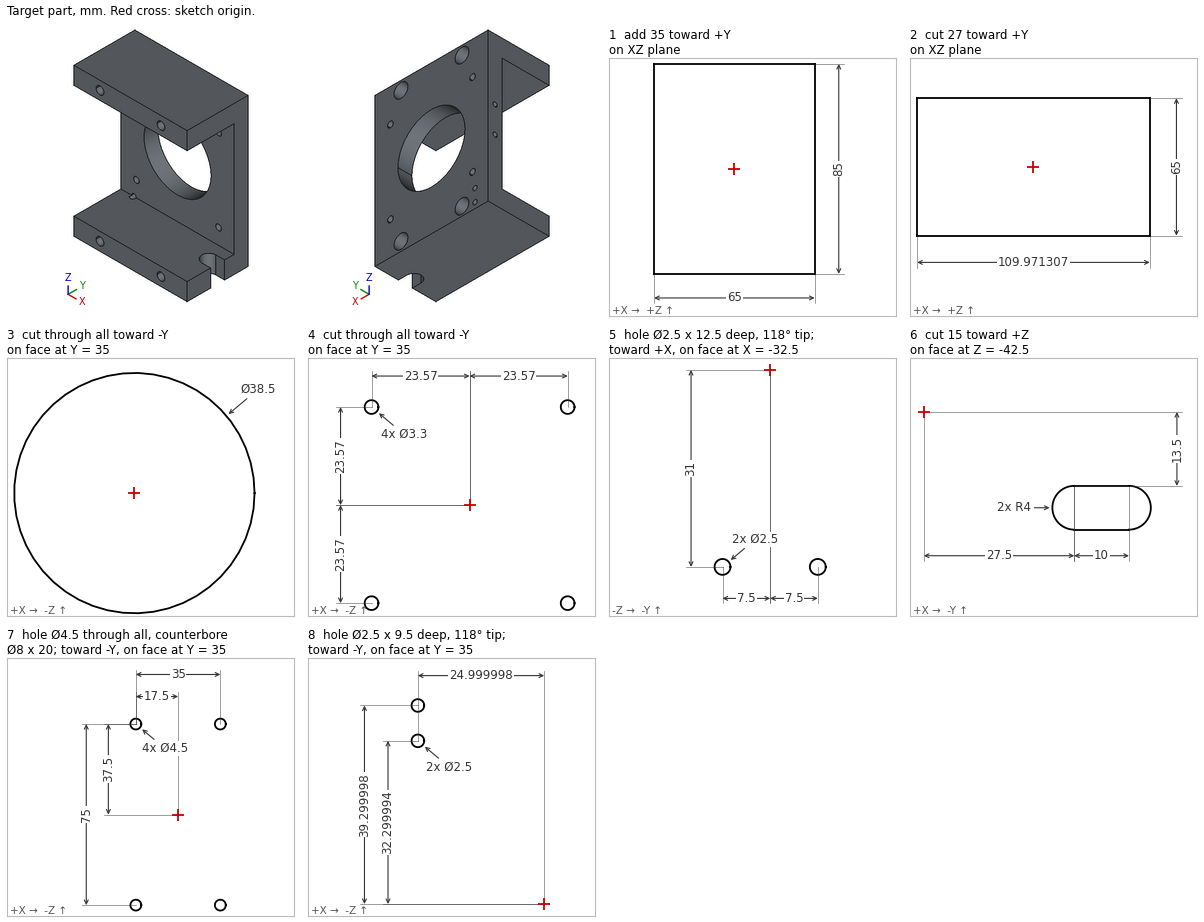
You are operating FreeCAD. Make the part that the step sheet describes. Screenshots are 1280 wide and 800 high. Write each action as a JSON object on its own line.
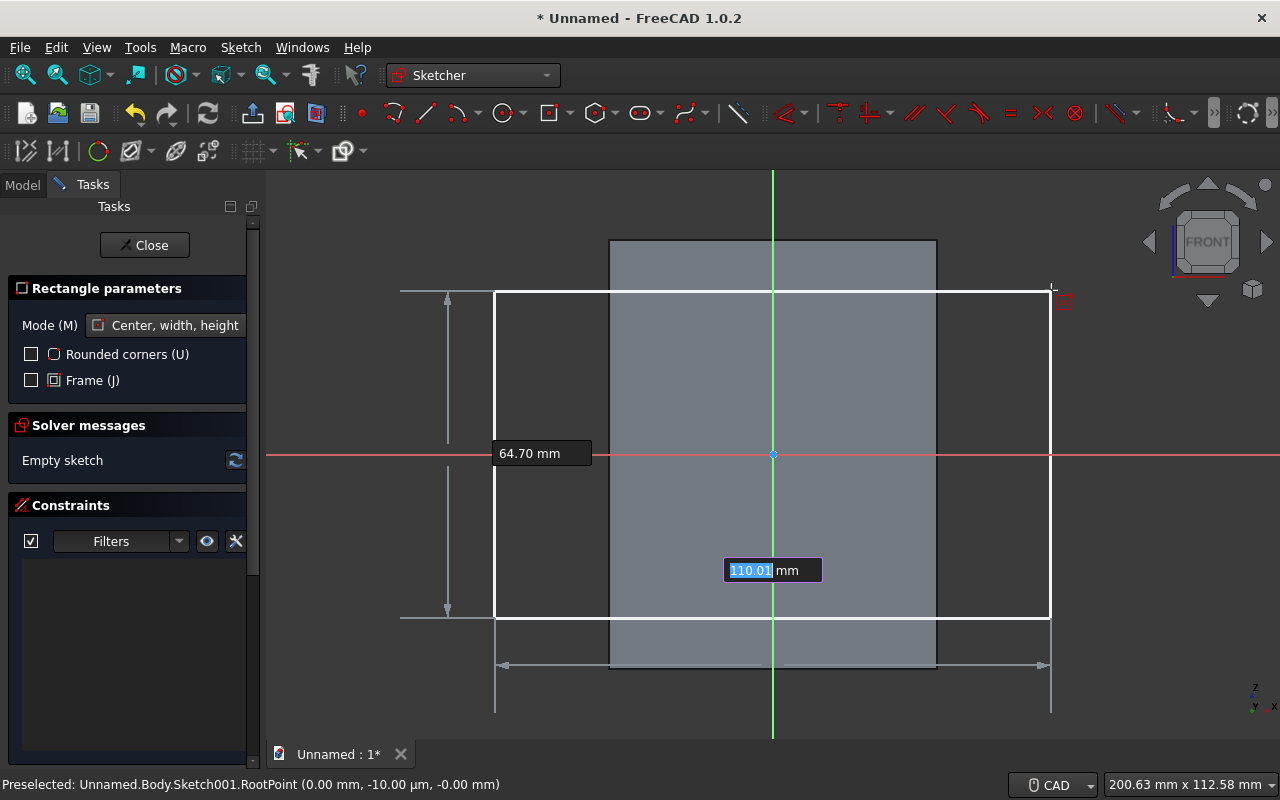
{"action": "type", "text": "109.971307"}
{"action": "key", "text": "Tab"}
{"action": "type", "text": "65"}
{"action": "key", "text": "Return"}
{"action": "key", "text": "Escape"}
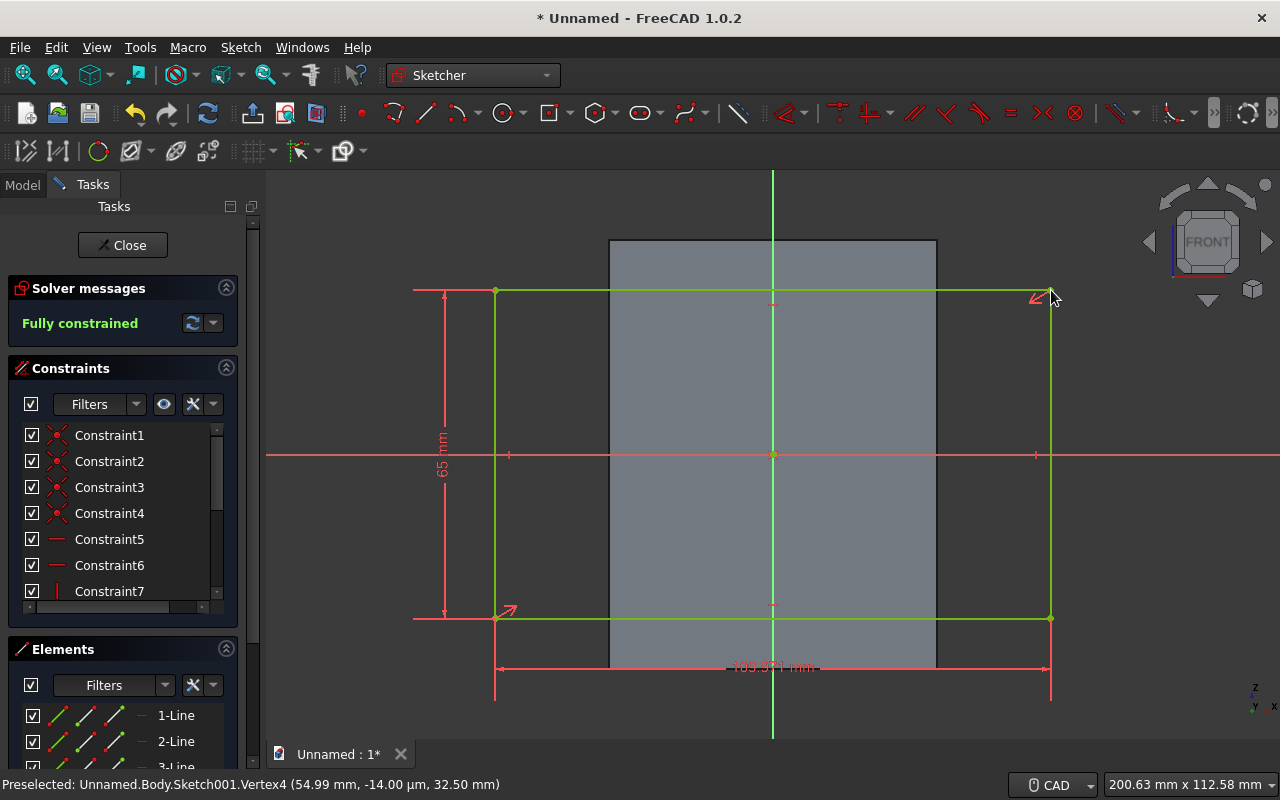
{"action": "left_click", "coordinate": [123, 245]}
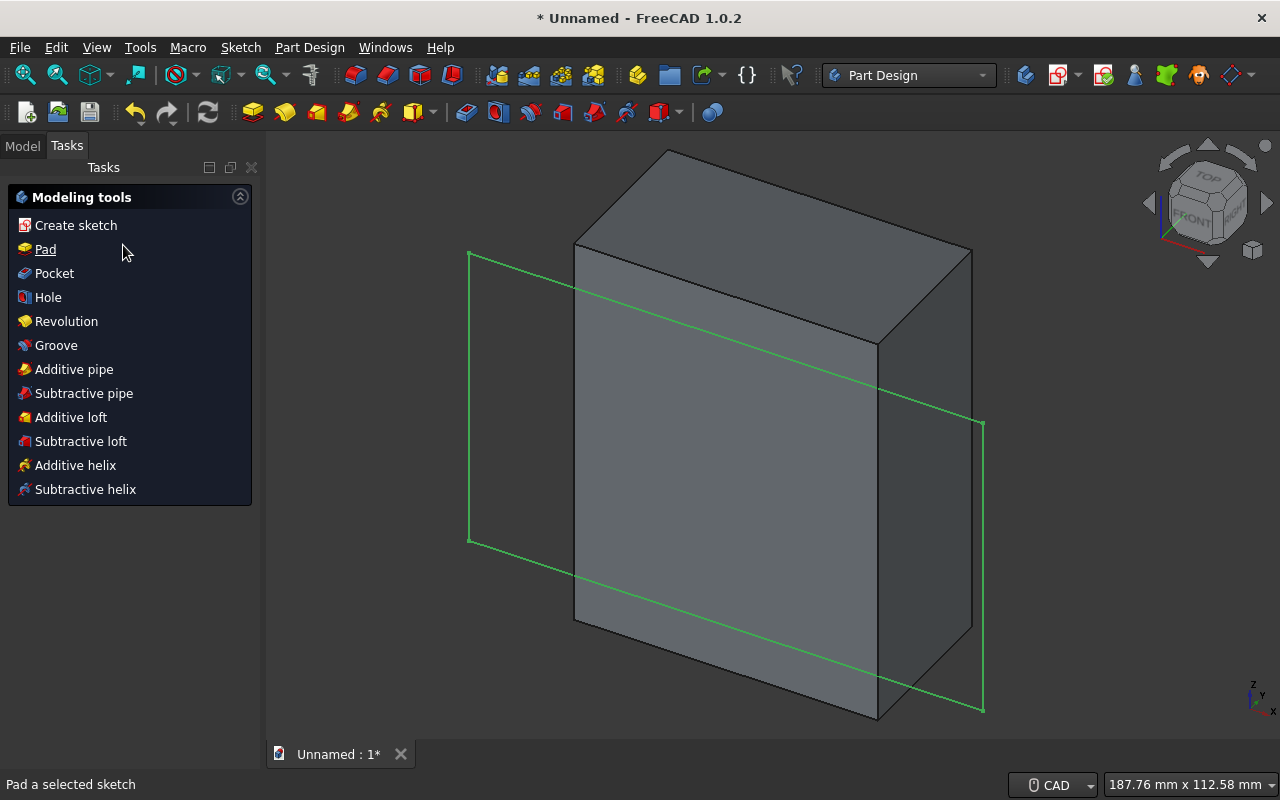
{"action": "left_click", "coordinate": [468, 112]}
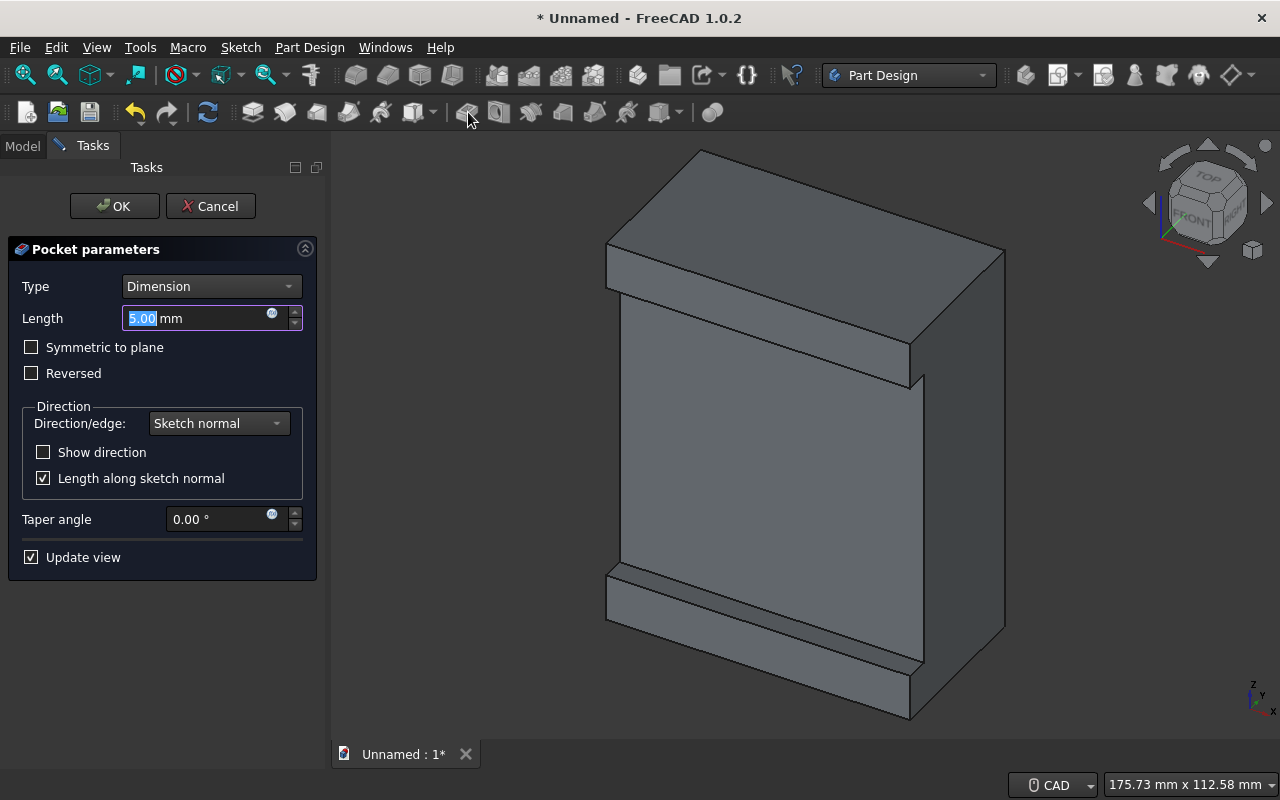
{"action": "type", "text": "27"}
{"action": "key", "text": "Tab"}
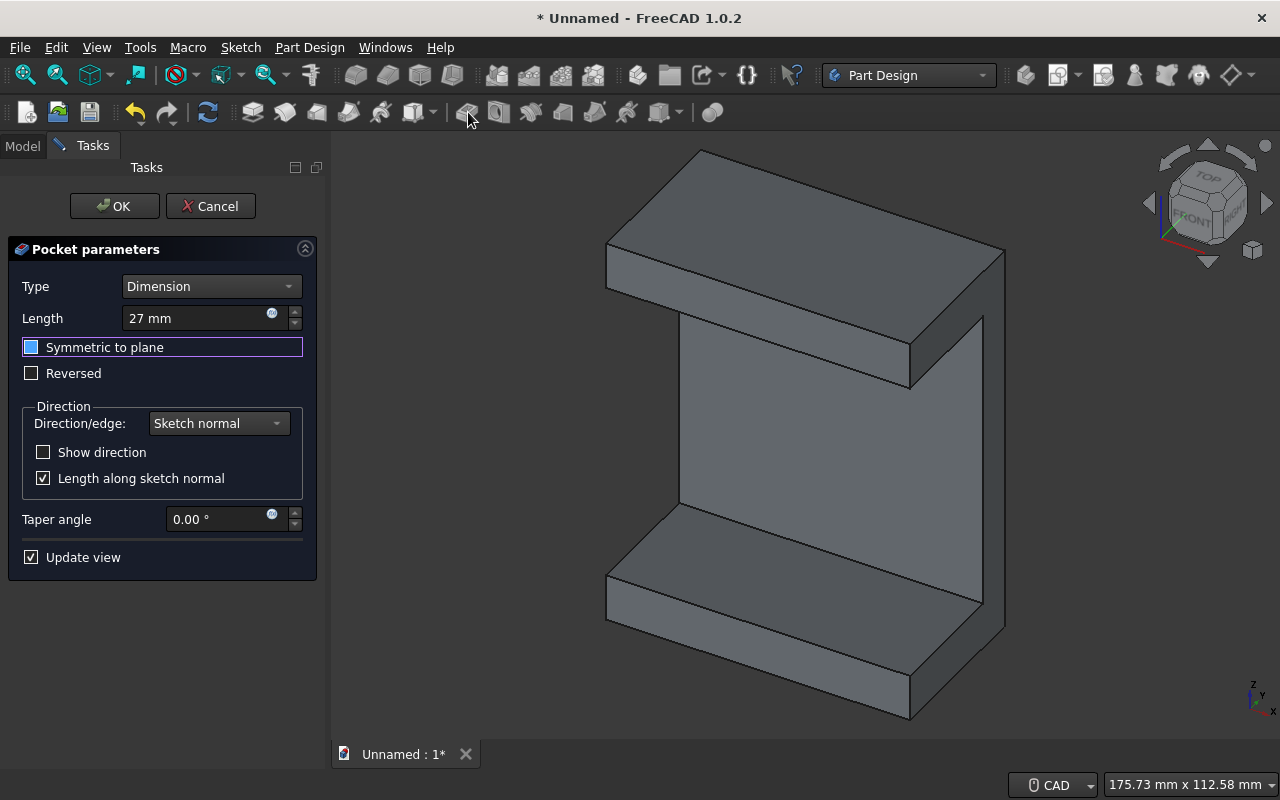
{"action": "left_click", "coordinate": [115, 206]}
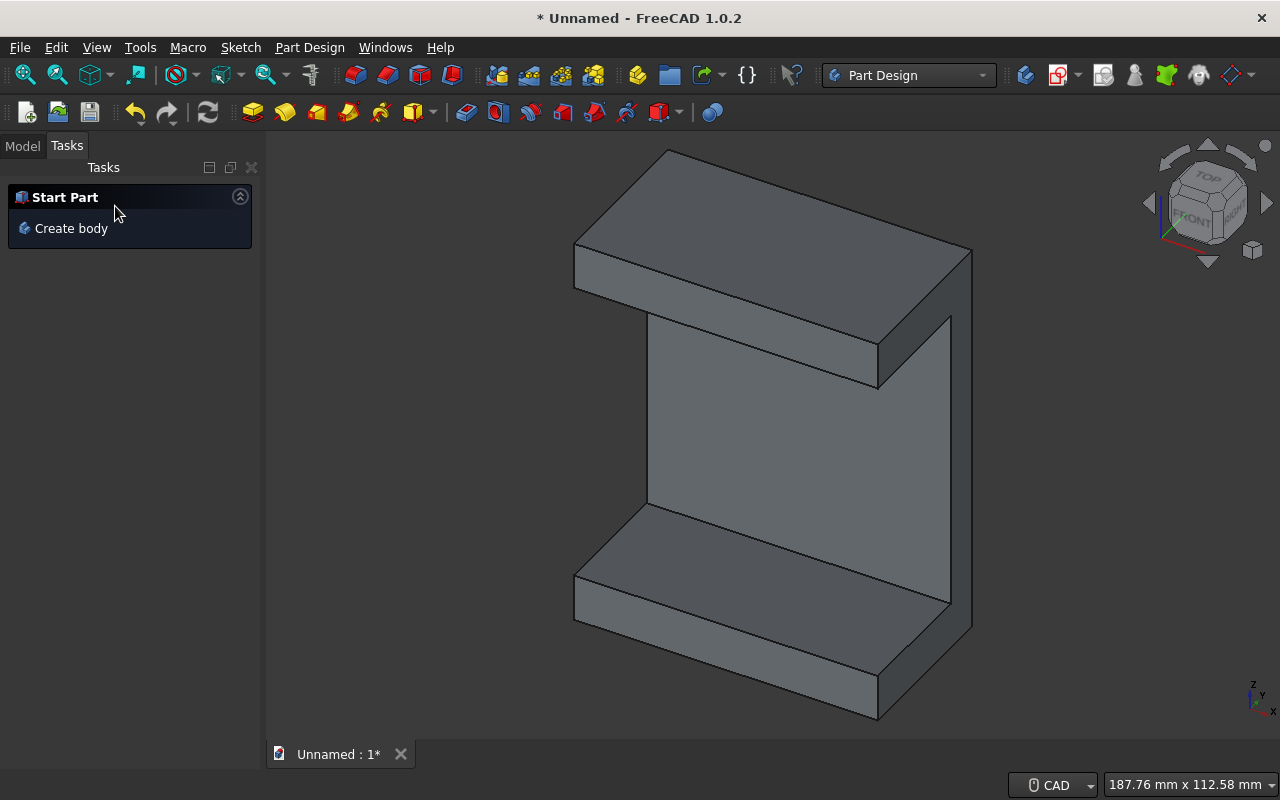
{"action": "key", "text": "4"}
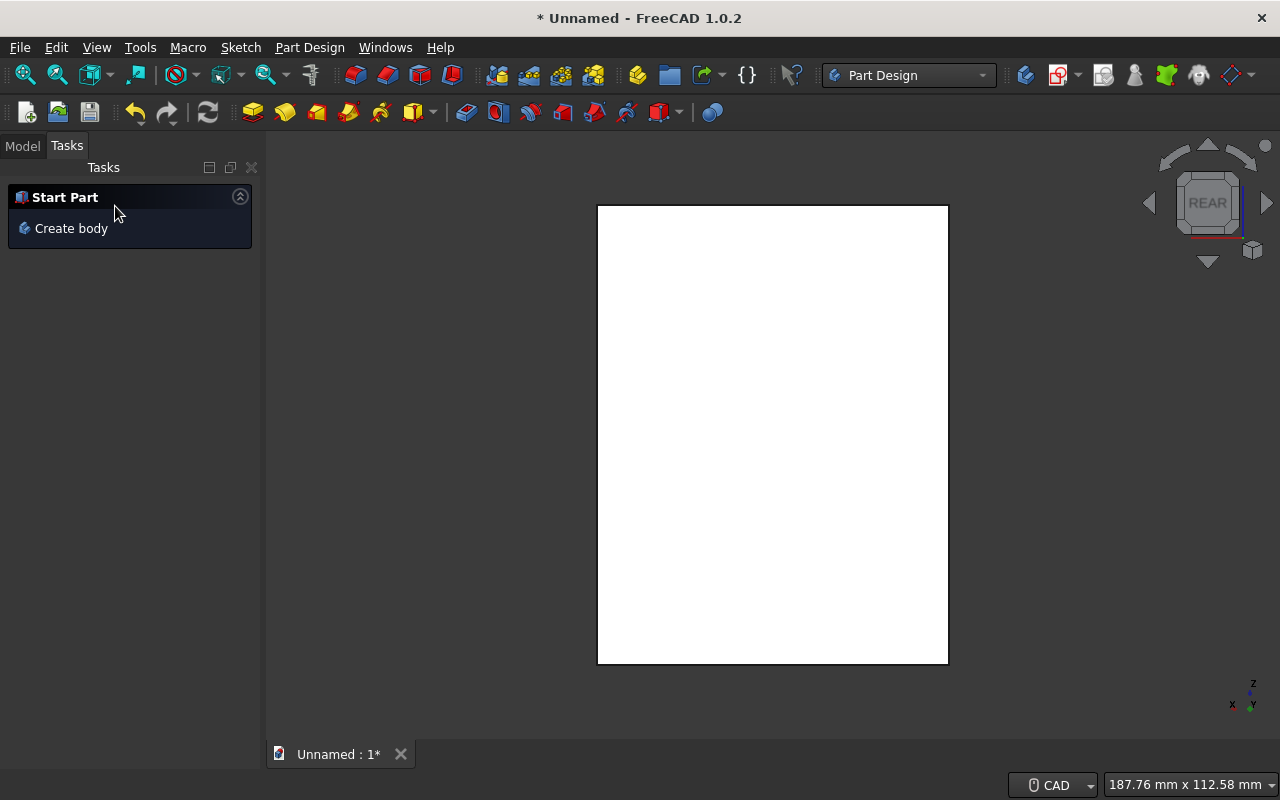
{"action": "left_click", "coordinate": [773, 434]}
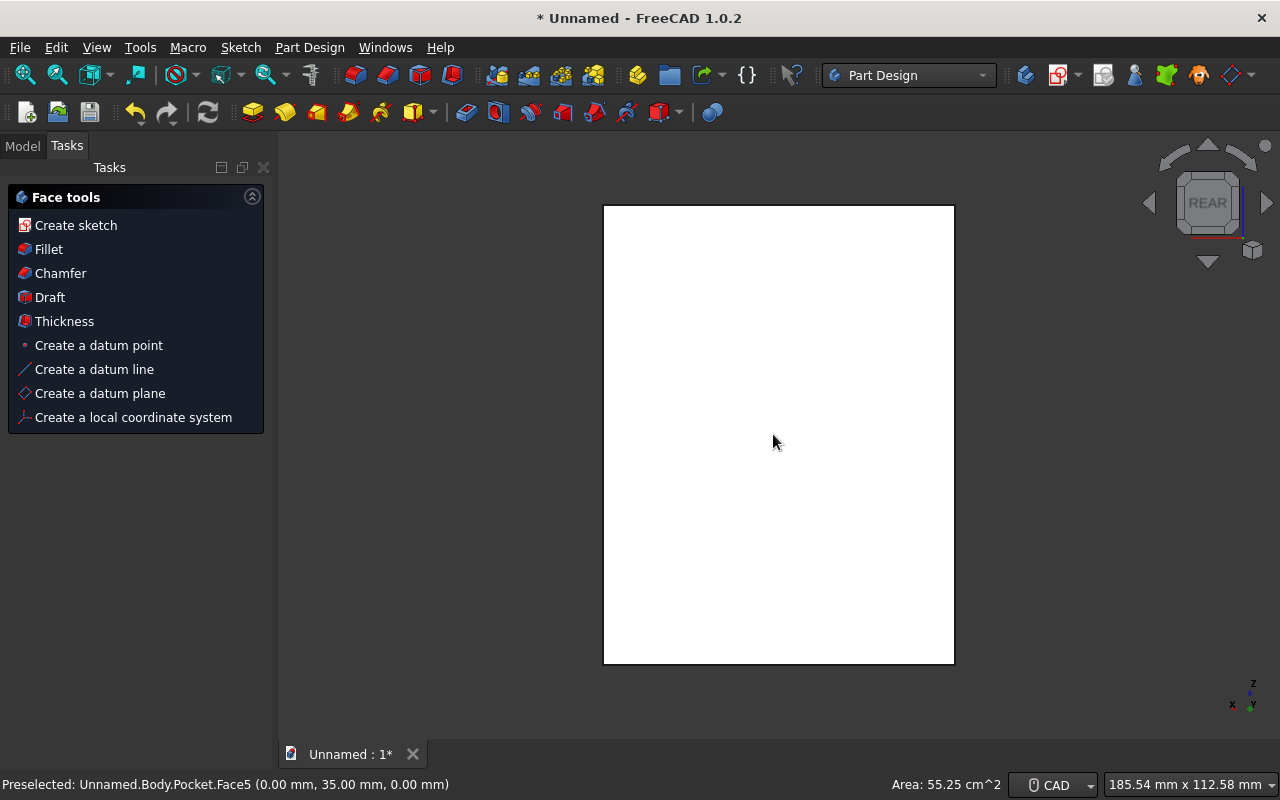
{"action": "left_click", "coordinate": [1058, 76]}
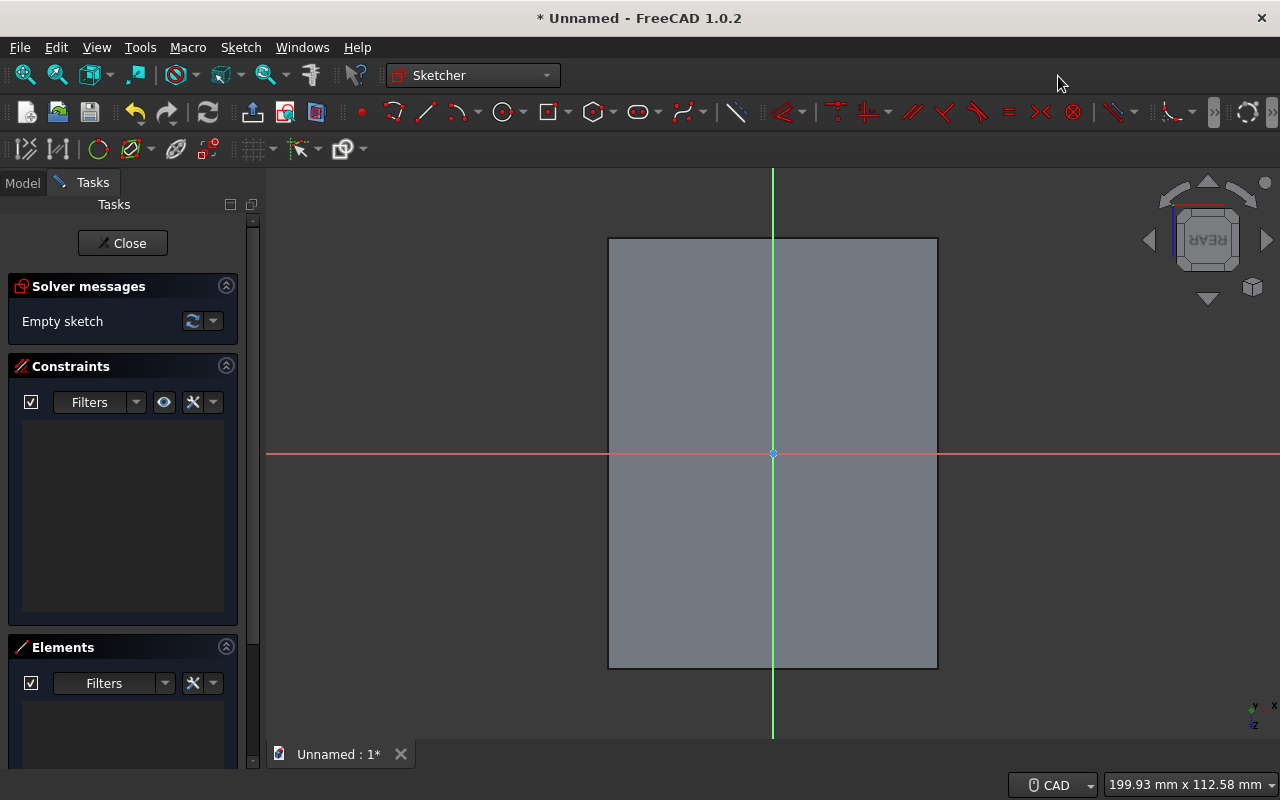
{"action": "scroll", "coordinate": [856, 454], "scroll_direction": "up", "scroll_amount": 3}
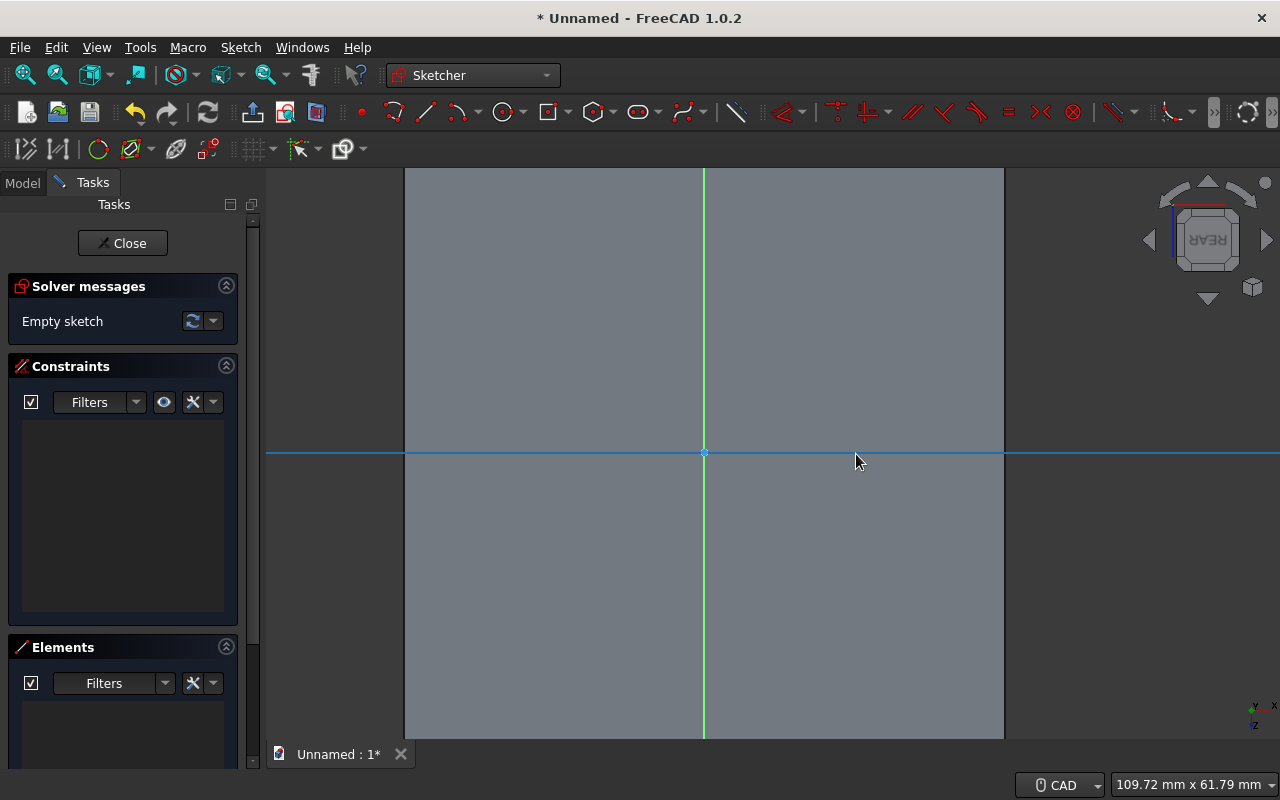
{"action": "left_click", "coordinate": [504, 112]}